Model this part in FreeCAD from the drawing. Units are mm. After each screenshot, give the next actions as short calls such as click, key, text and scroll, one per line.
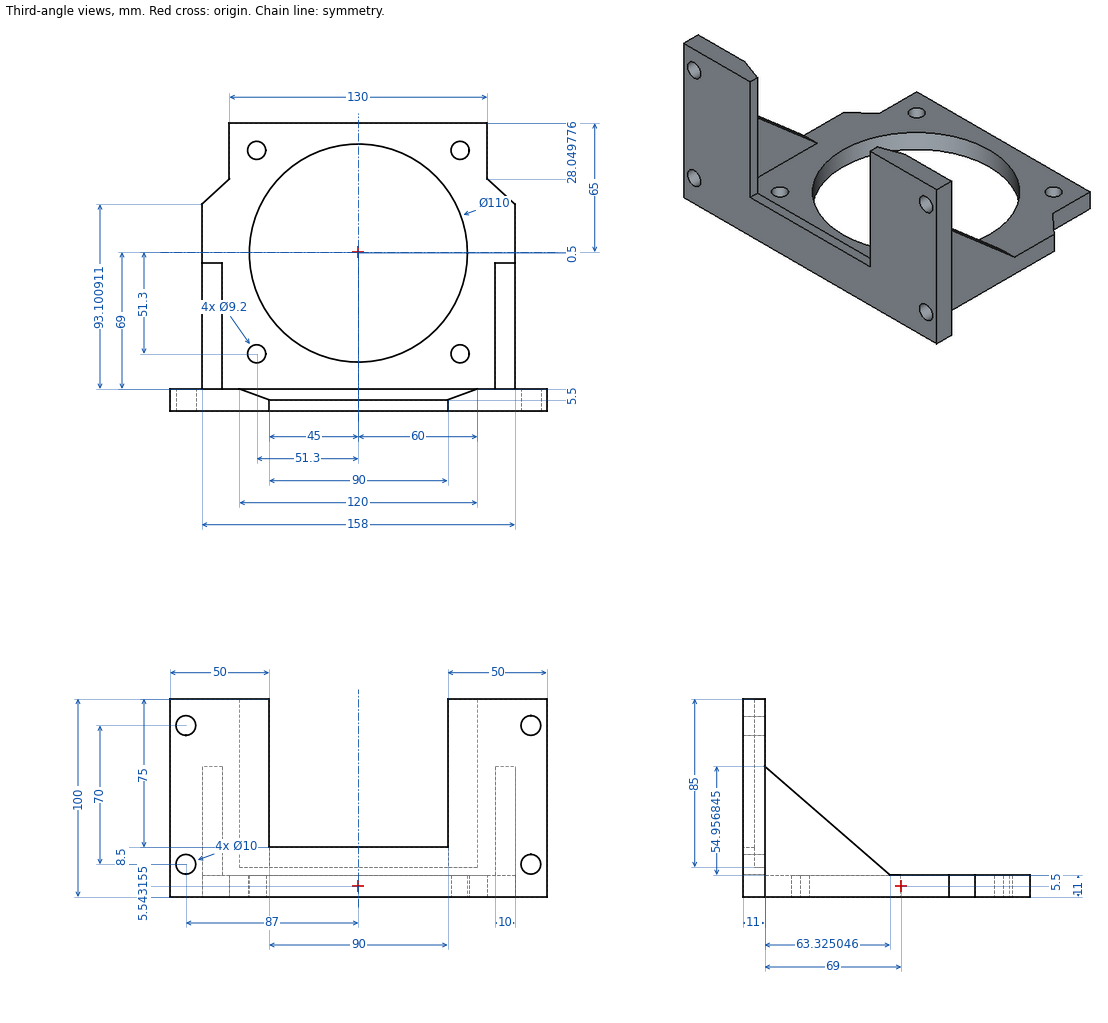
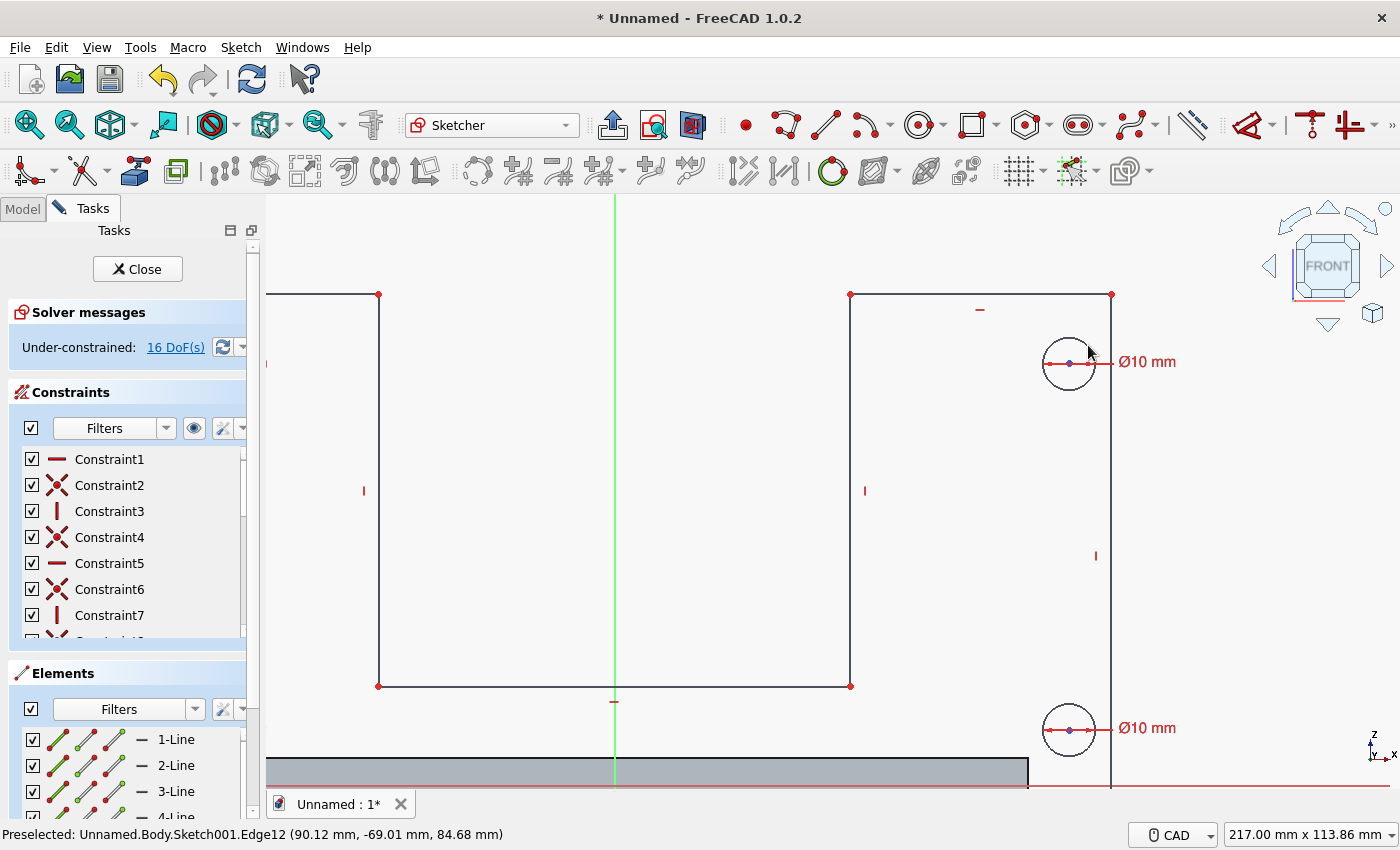
scroll(1069, 364, down, 2)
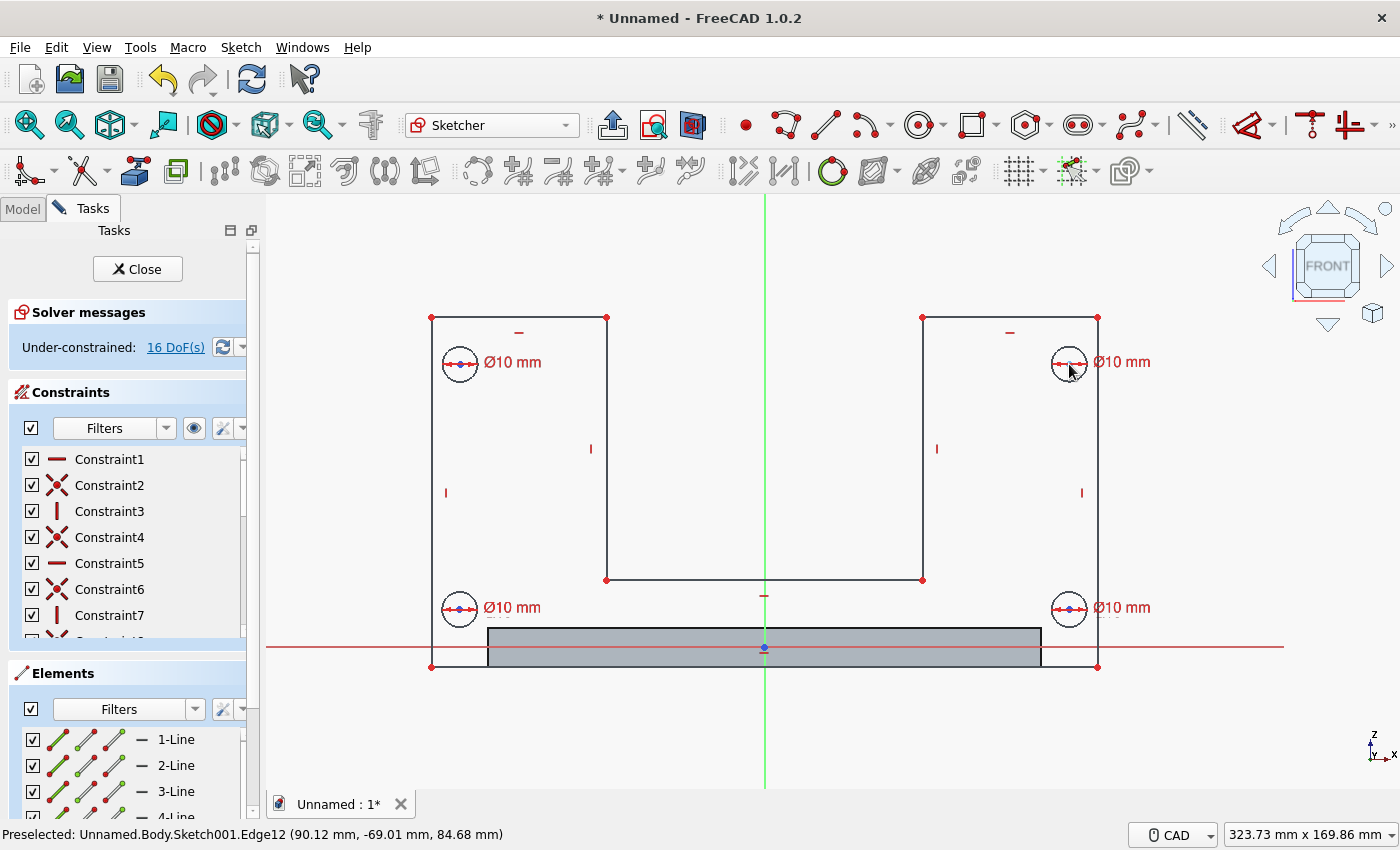
click(460, 610)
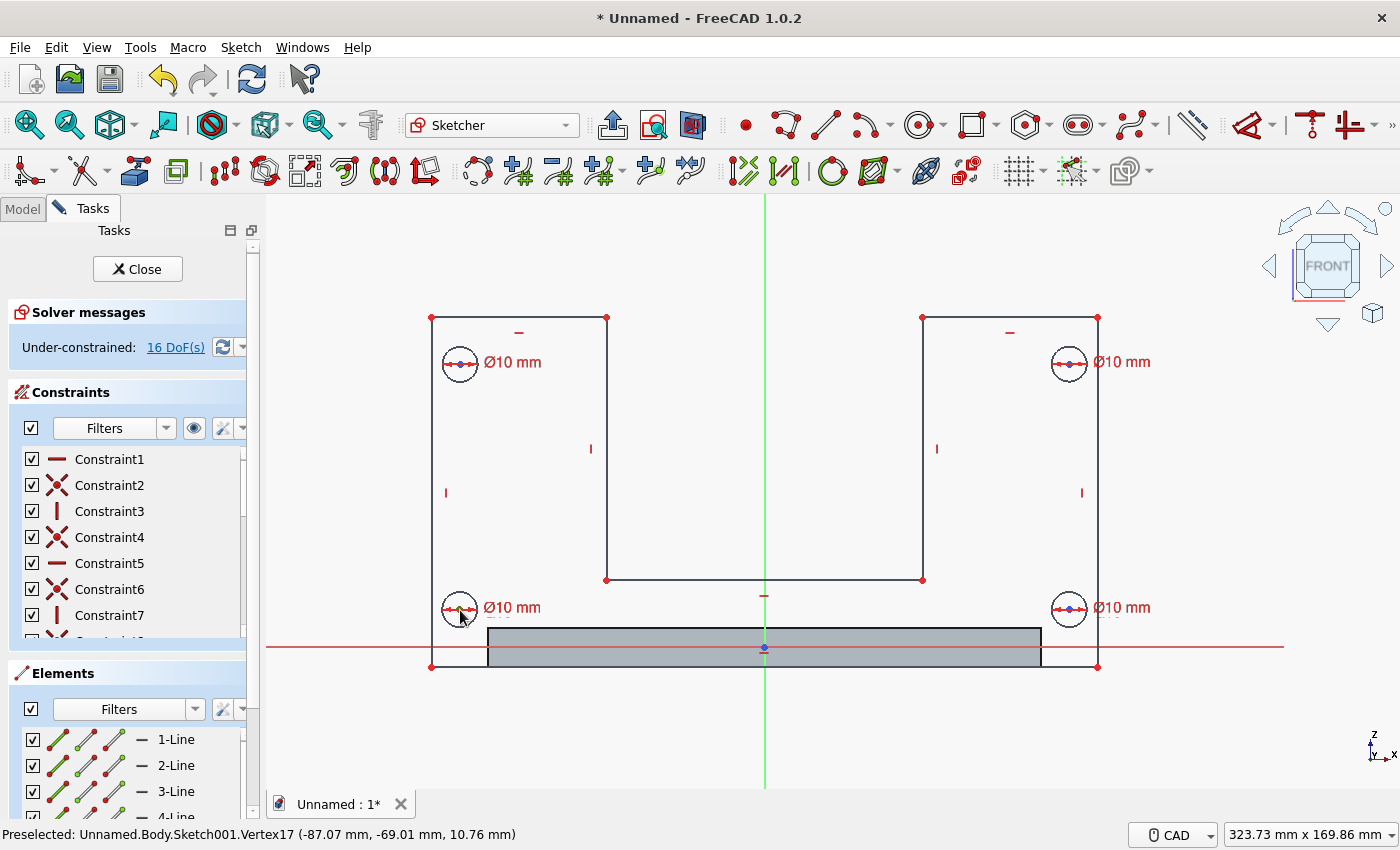
click(460, 364)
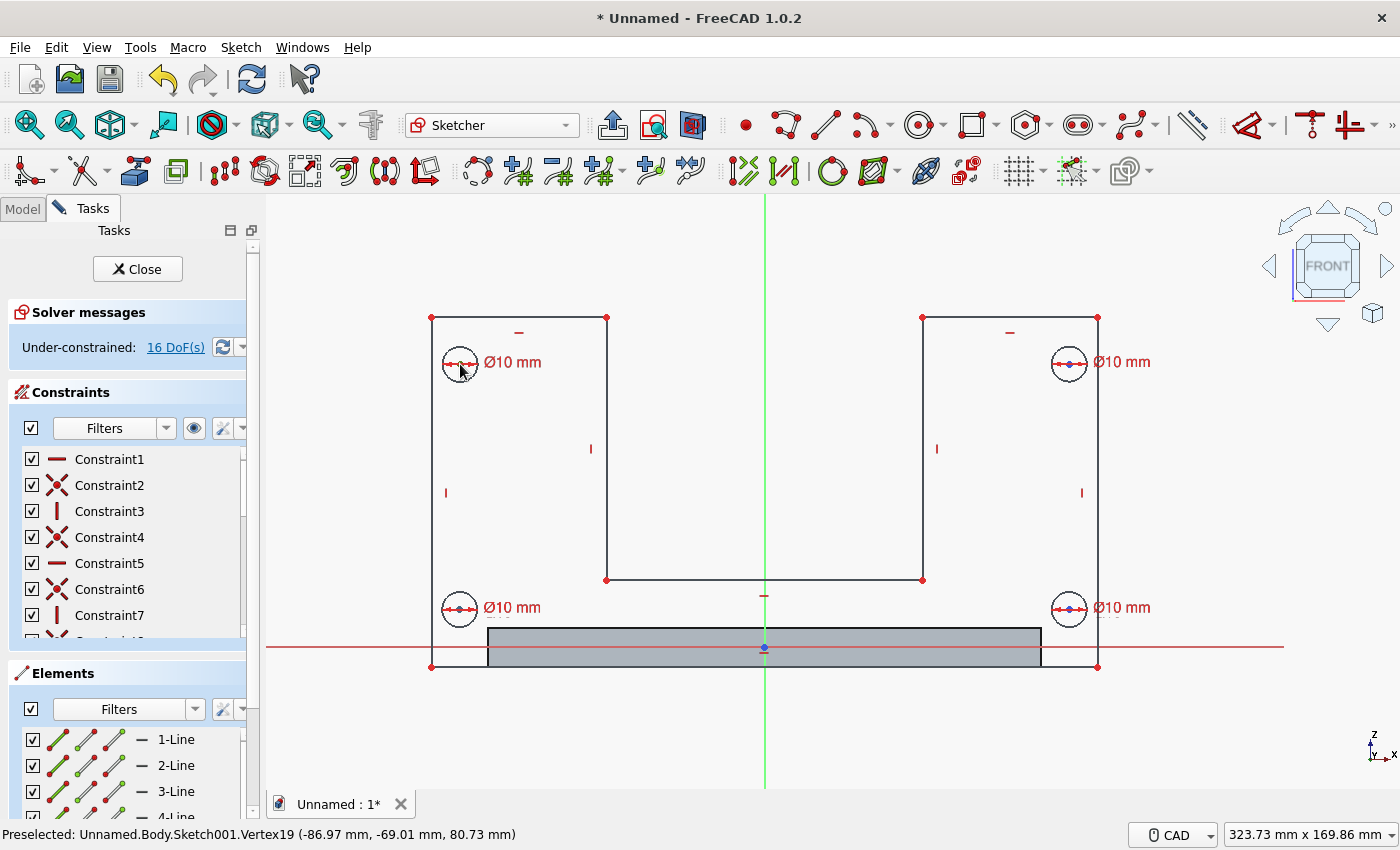
click(1376, 126)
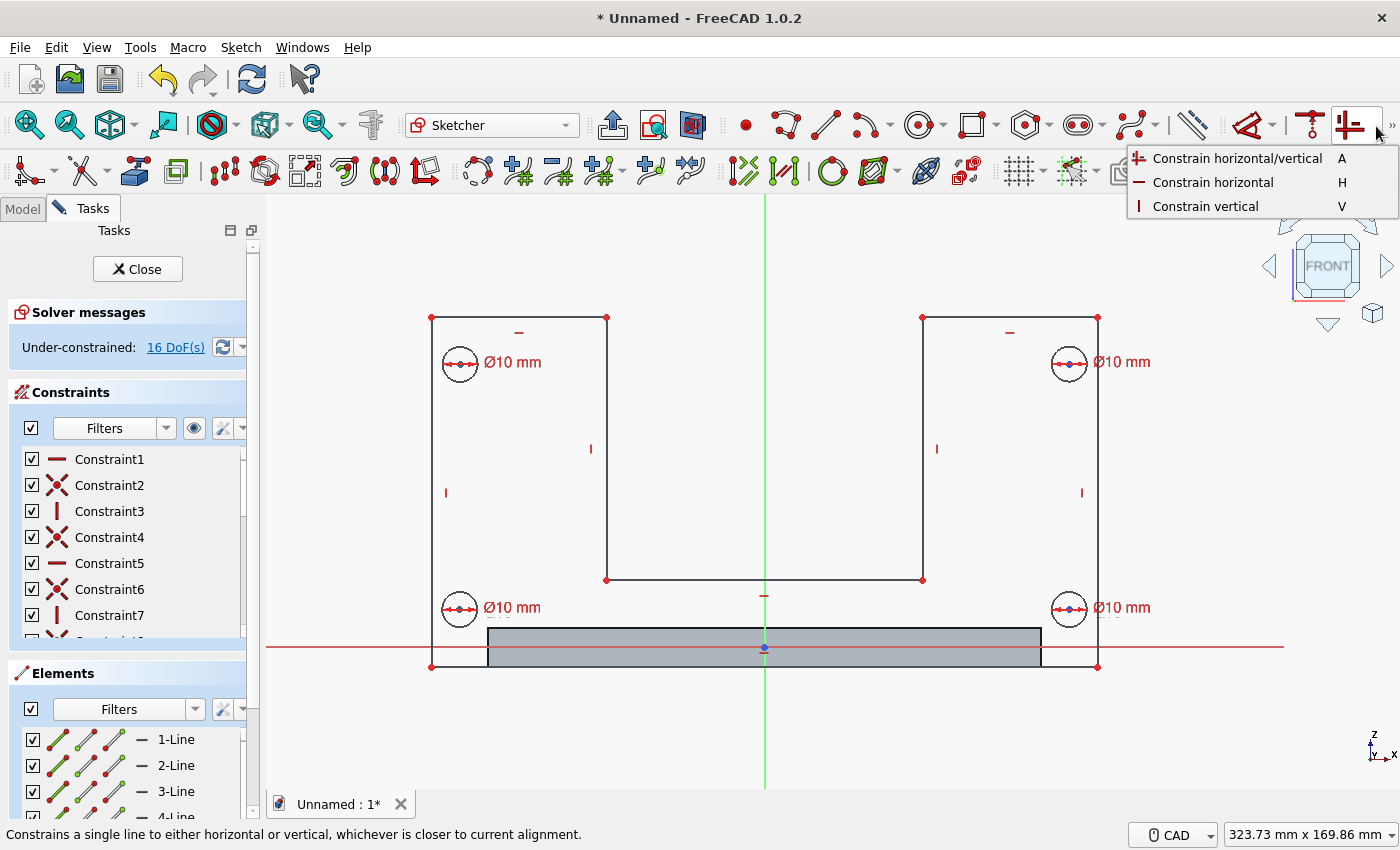
click(1263, 206)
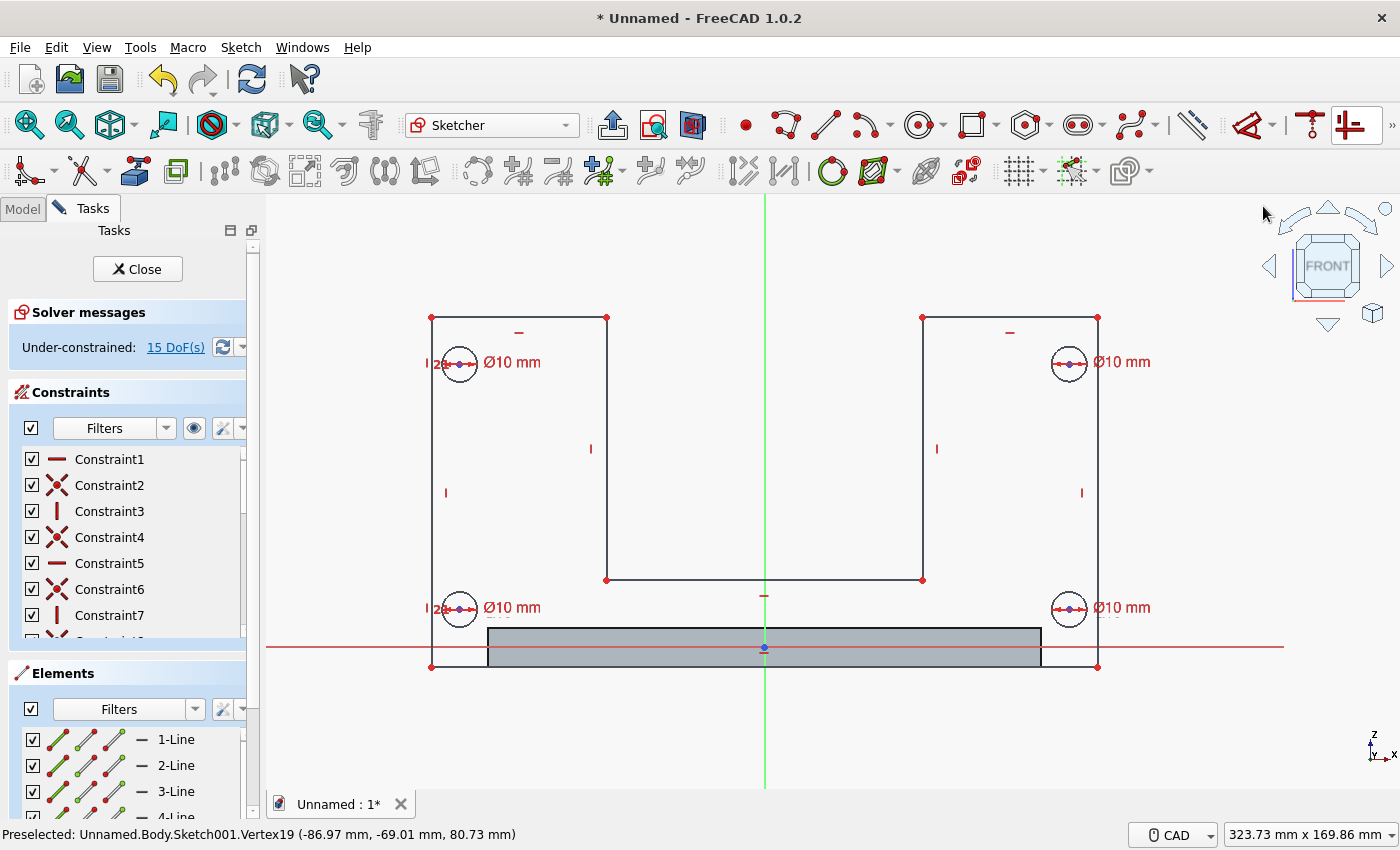
click(1069, 610)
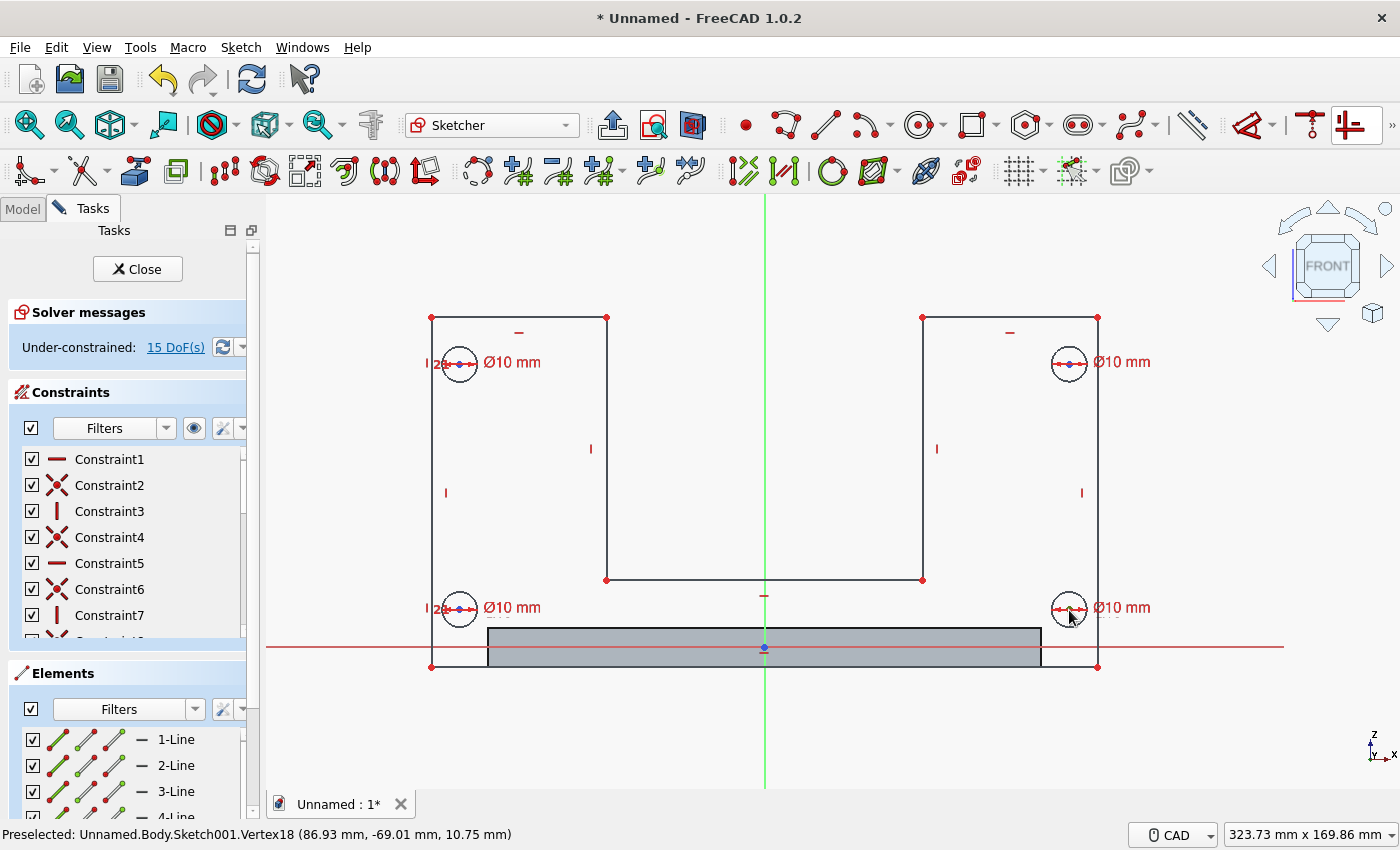
click(1069, 364)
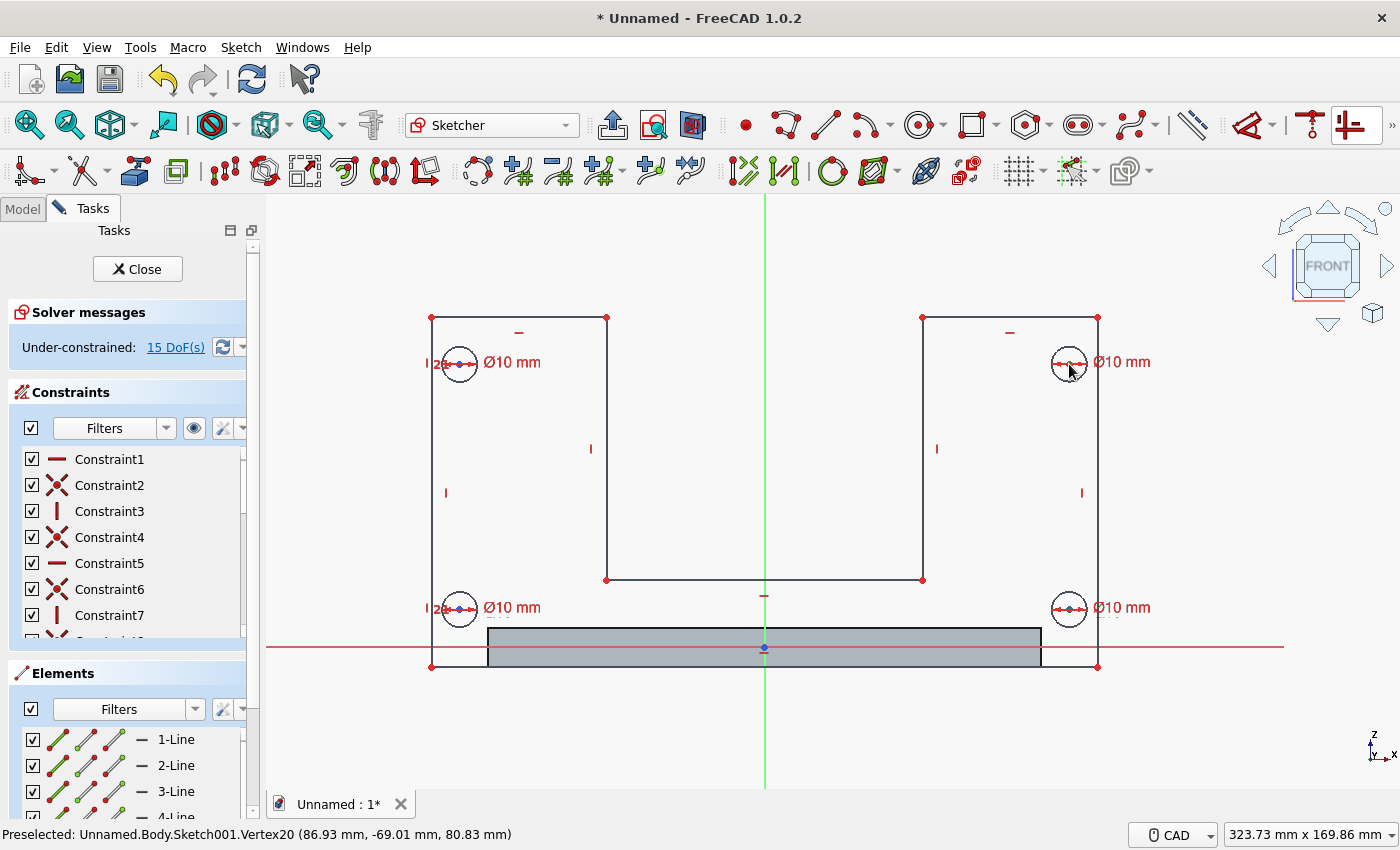
click(1376, 126)